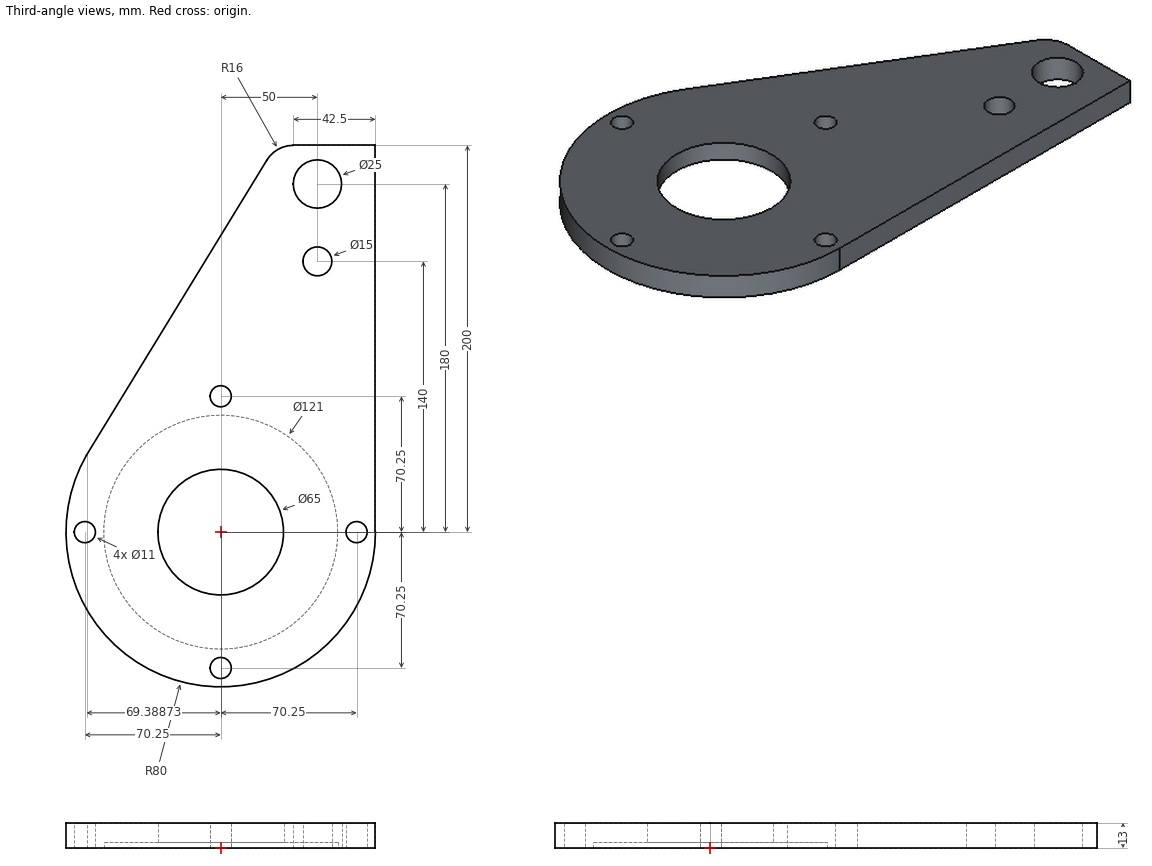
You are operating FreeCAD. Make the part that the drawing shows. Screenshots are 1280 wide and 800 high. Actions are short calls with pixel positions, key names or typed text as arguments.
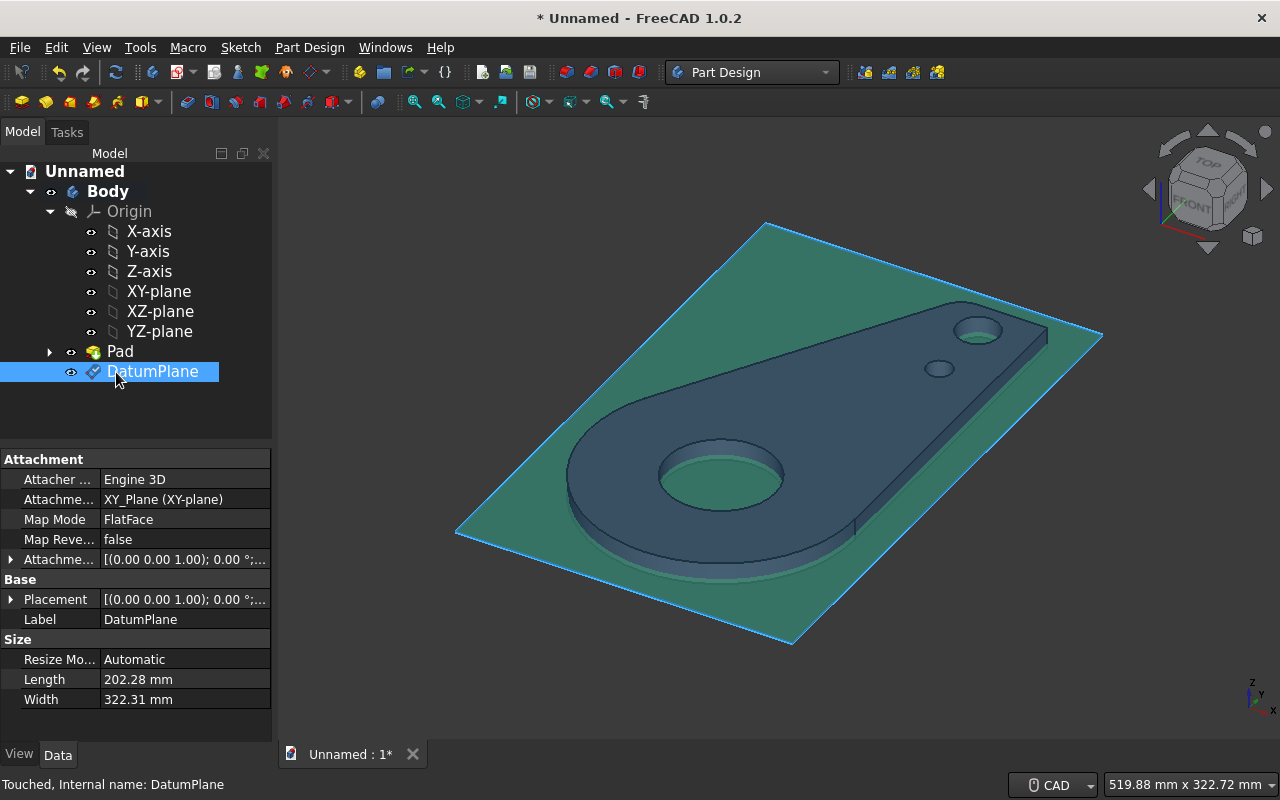
click(178, 72)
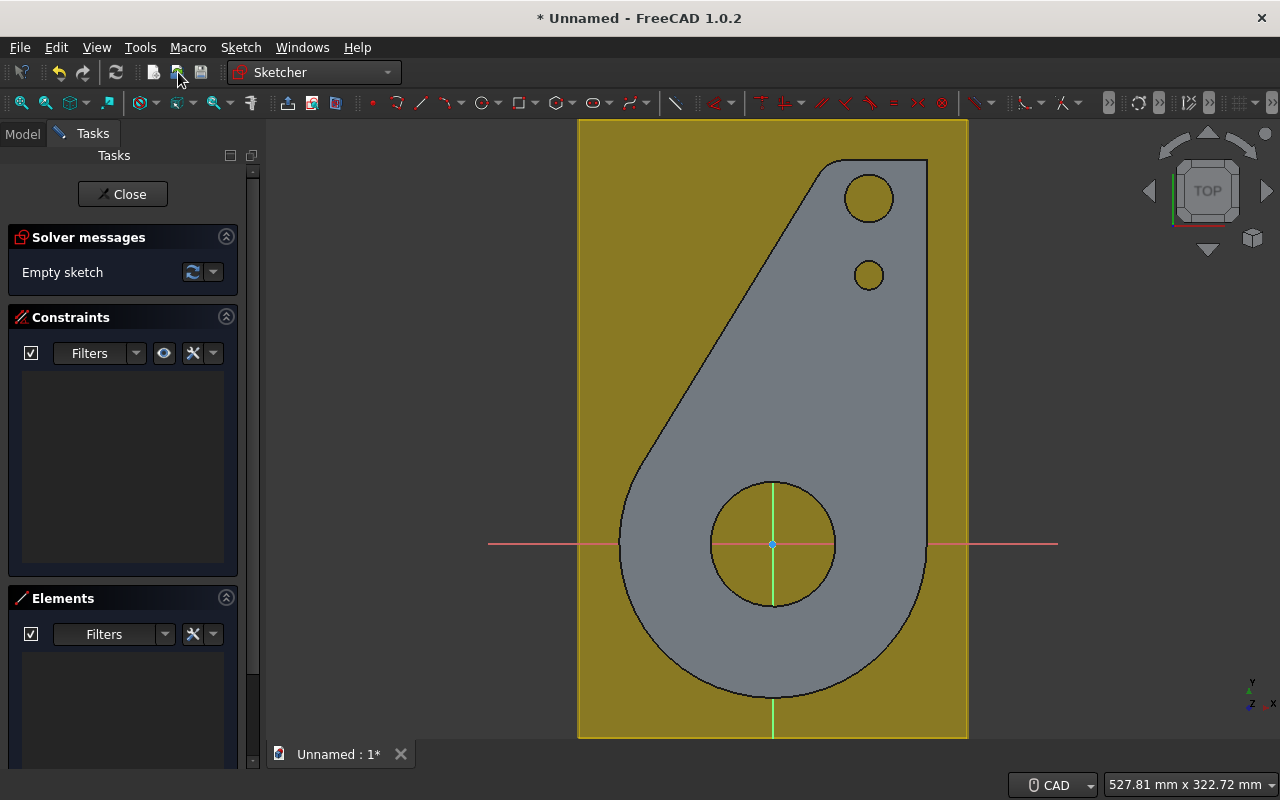
click(336, 104)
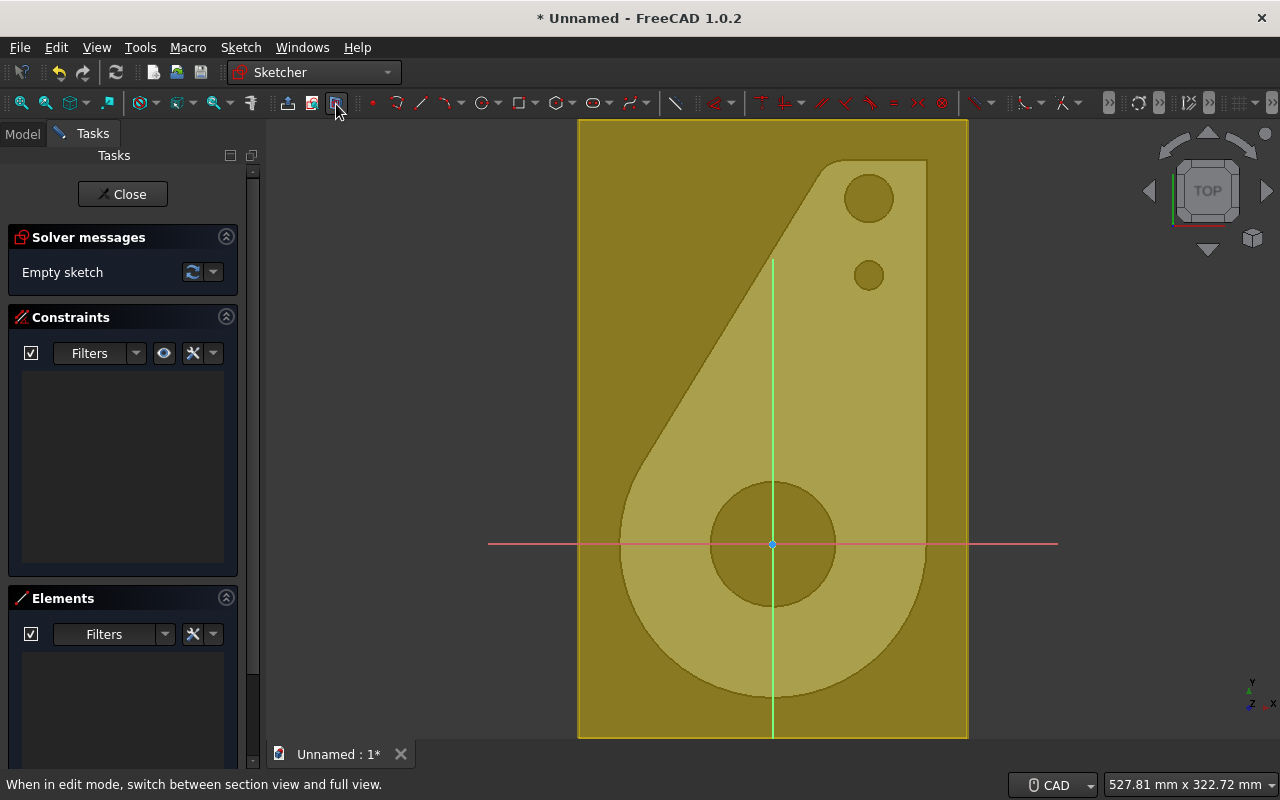
scroll(856, 685, up, 3)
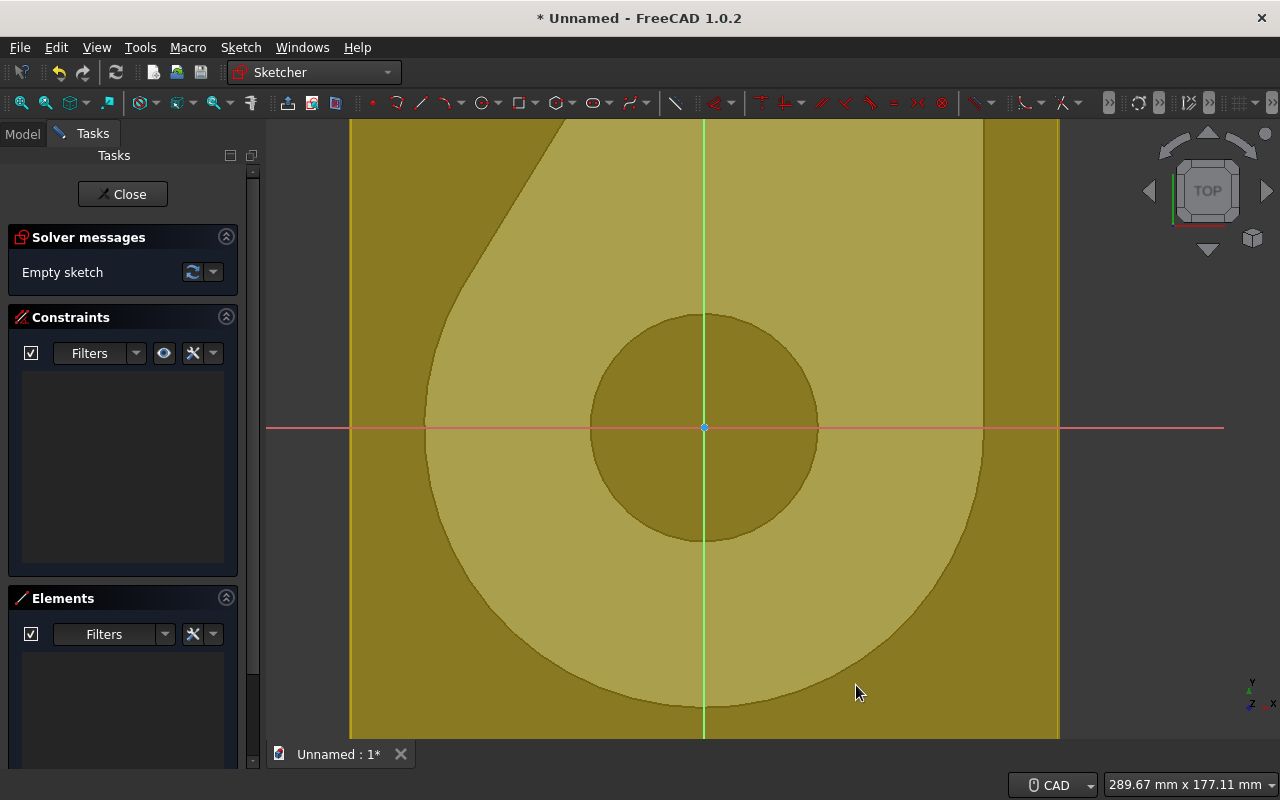
click(482, 104)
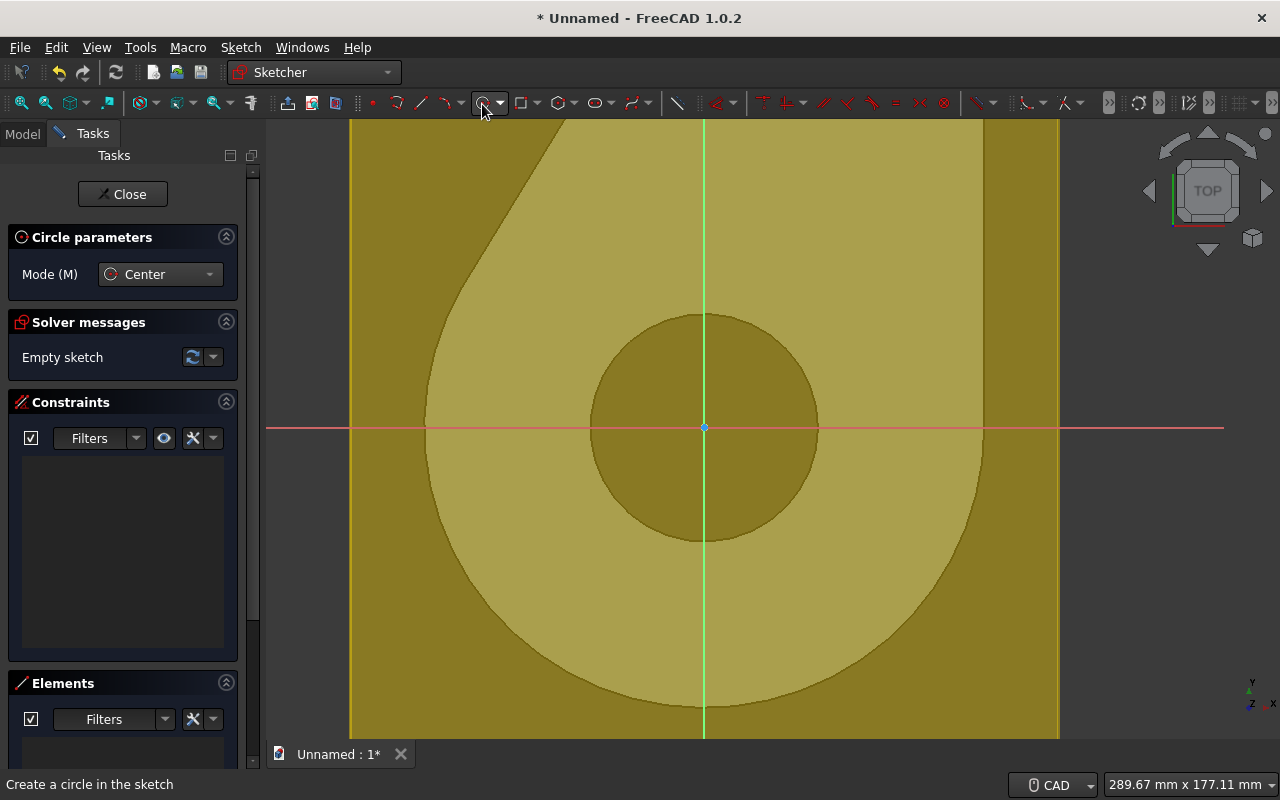
click(704, 428)
click(854, 278)
key(Escape)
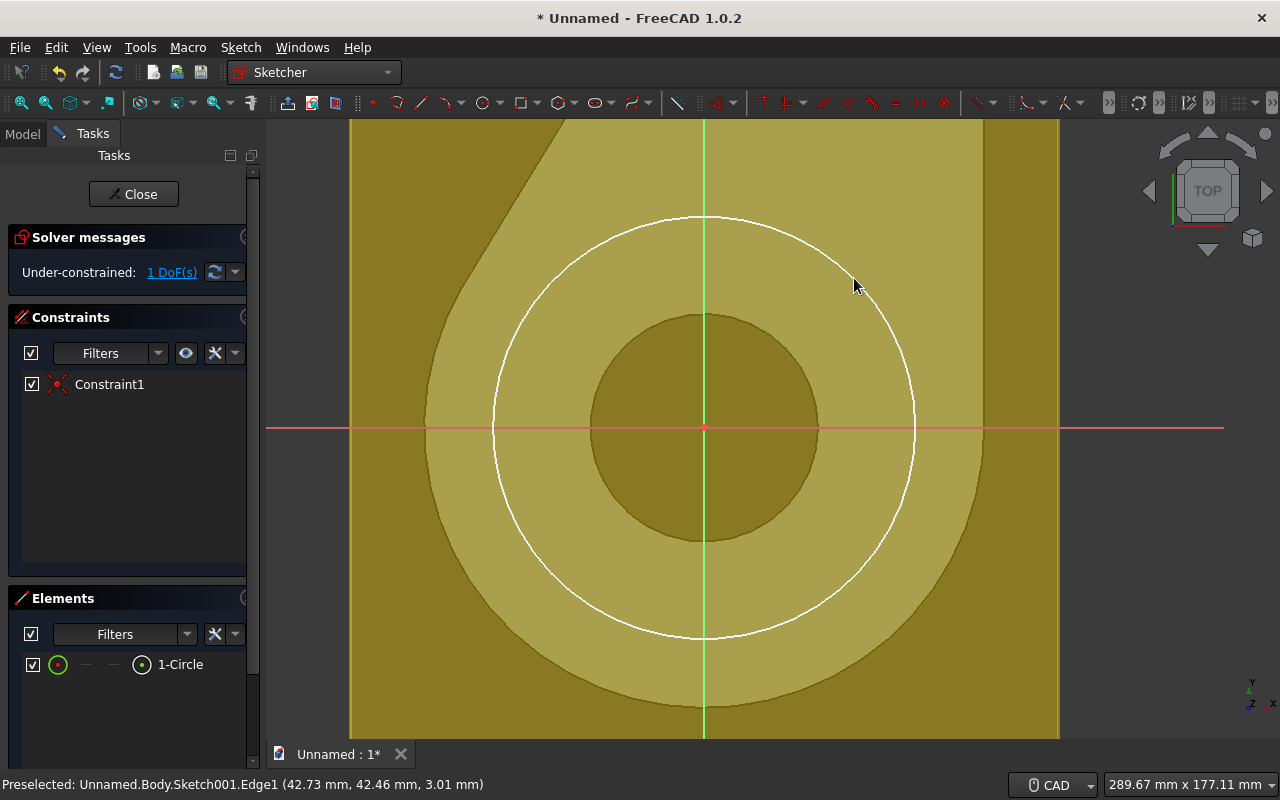
click(716, 104)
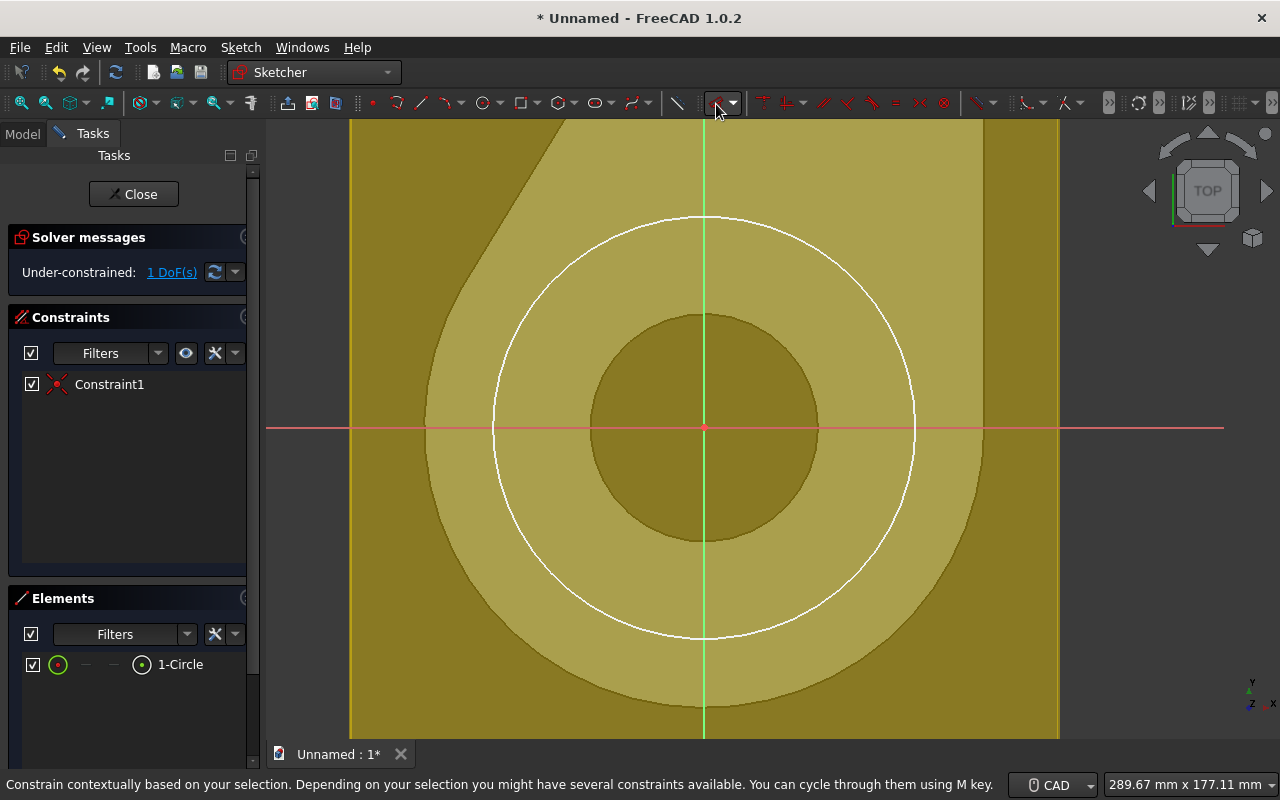
click(853, 278)
click(876, 255)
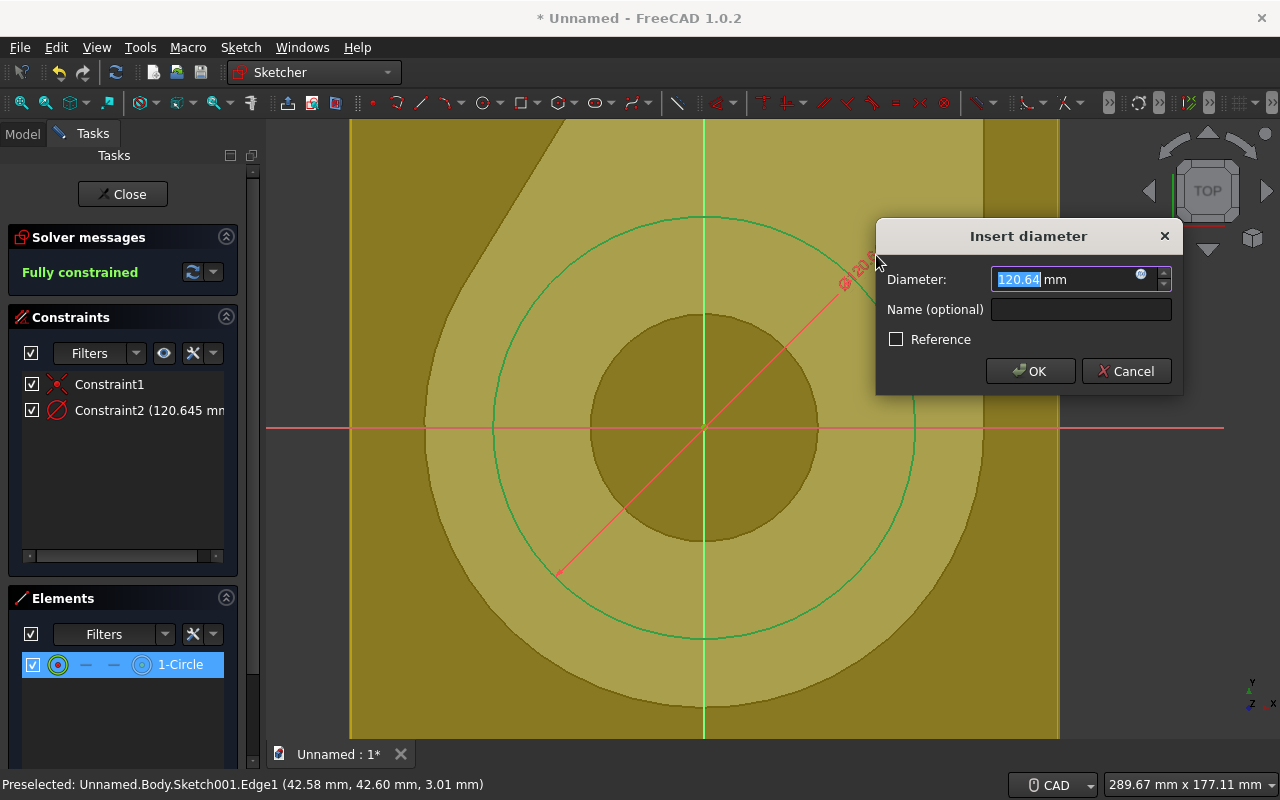
text(121)
key(Return)
key(Escape)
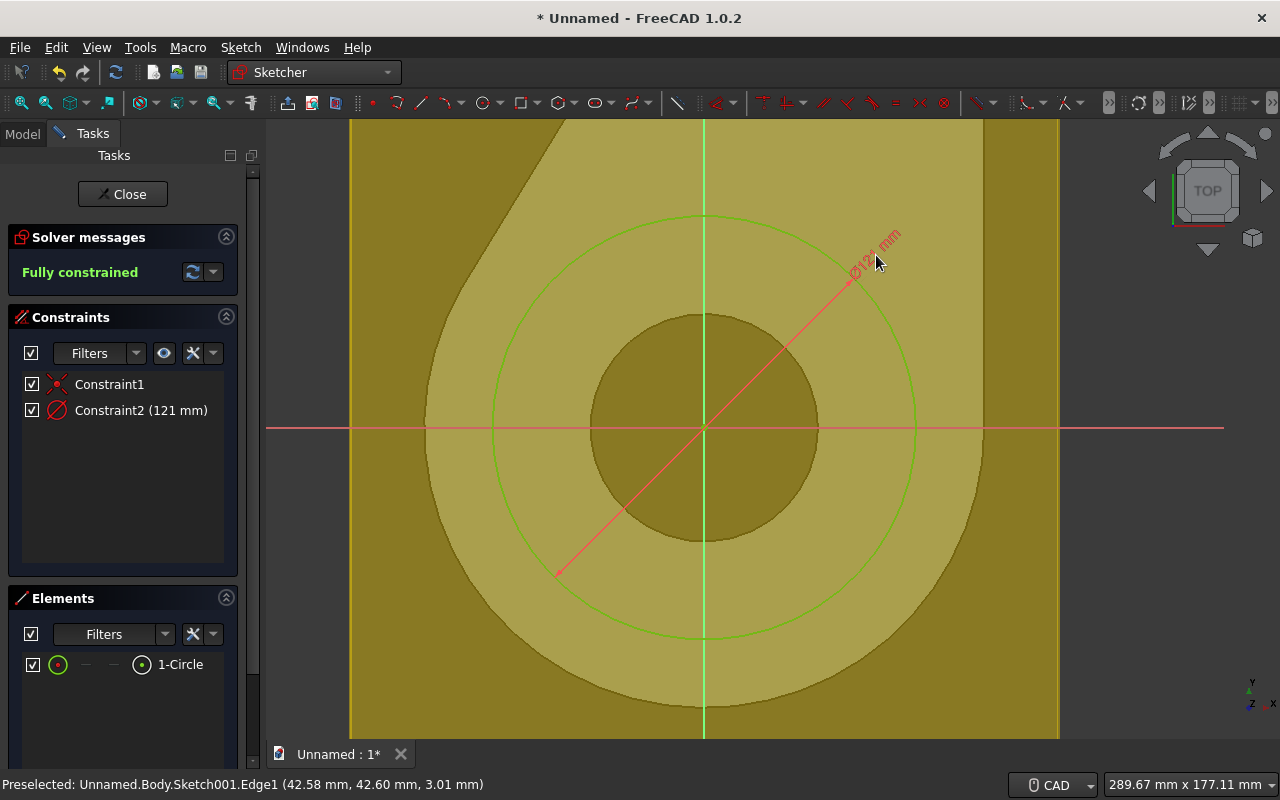
click(123, 194)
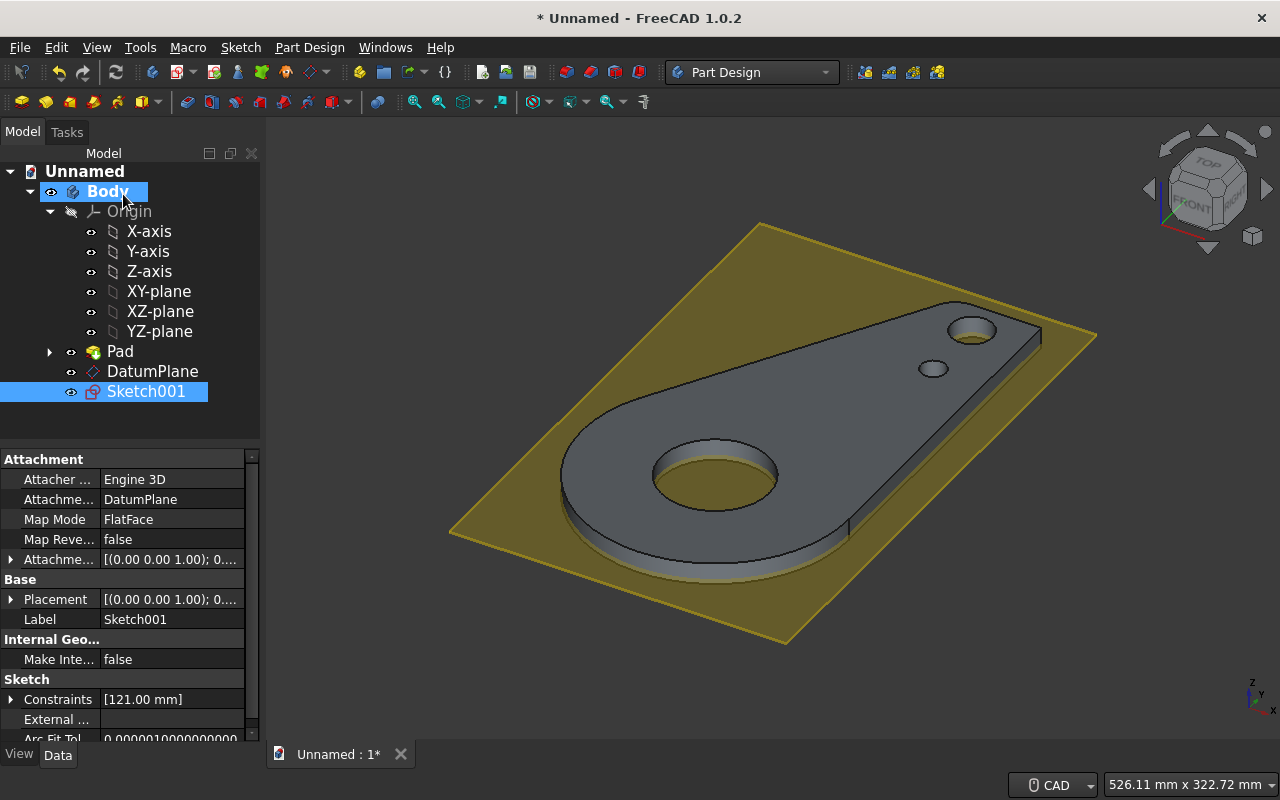
click(188, 102)